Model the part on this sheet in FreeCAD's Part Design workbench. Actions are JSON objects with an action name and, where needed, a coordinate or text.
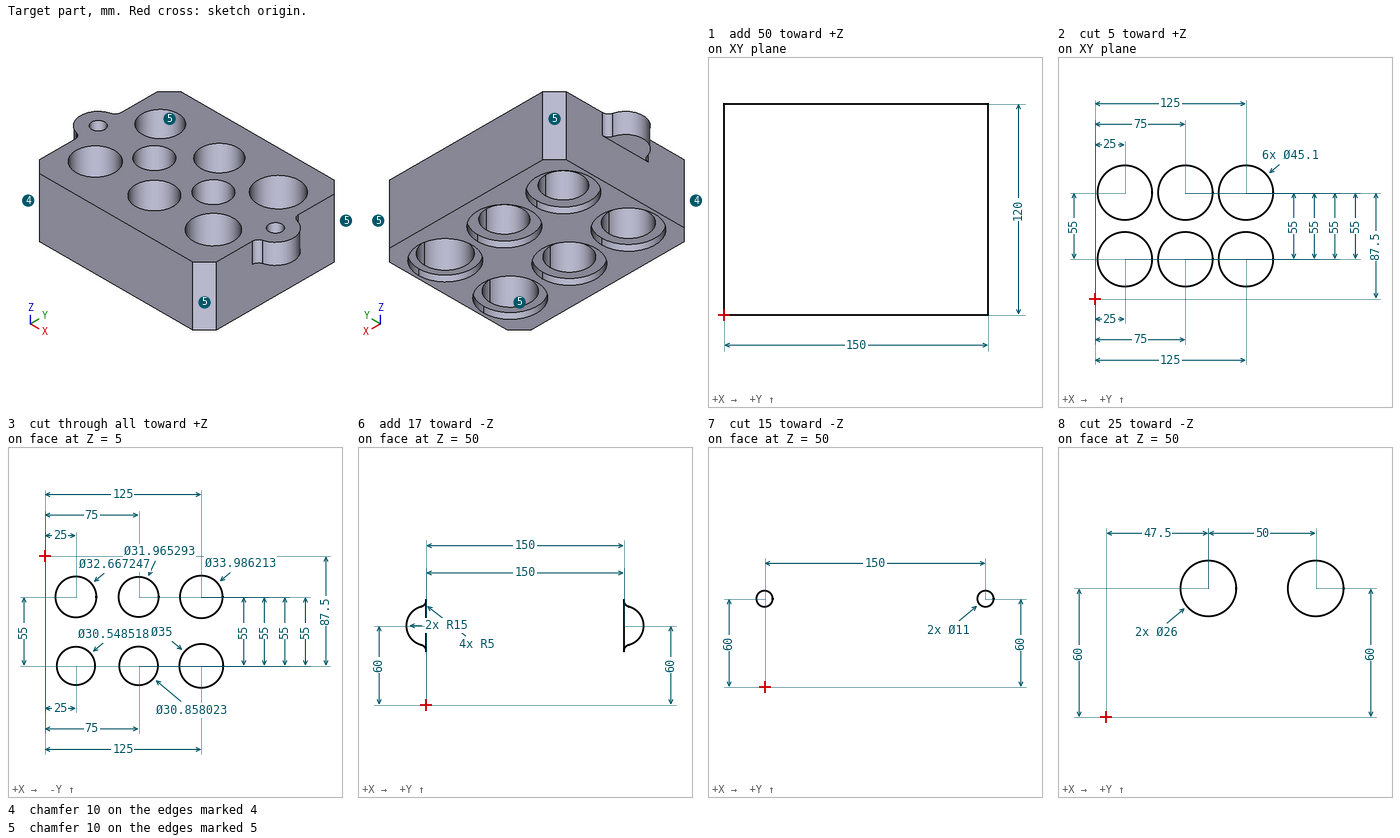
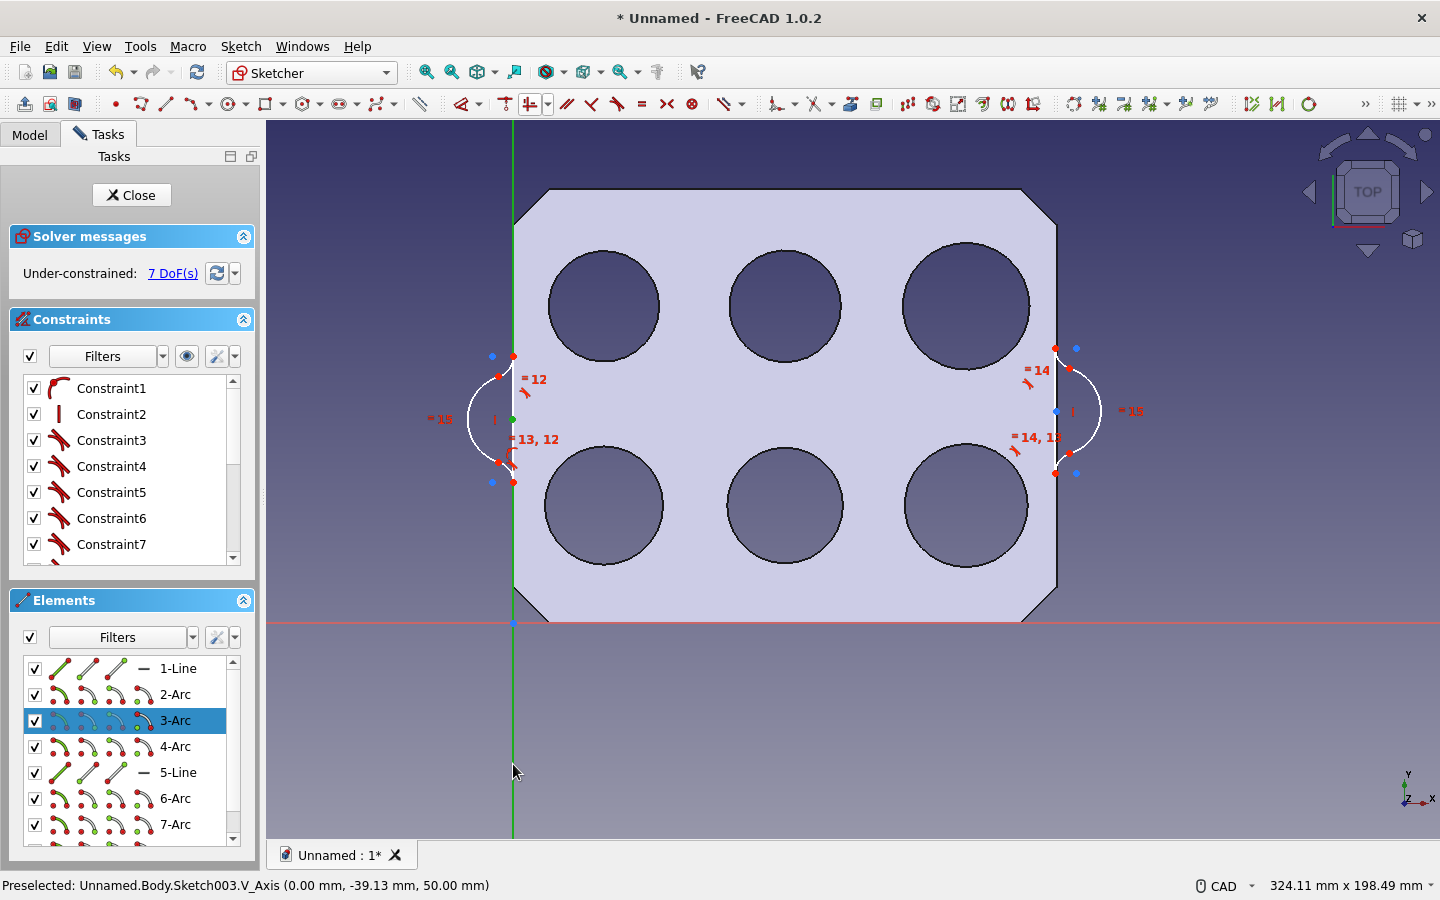
{"action": "left_click", "coordinate": [505, 104]}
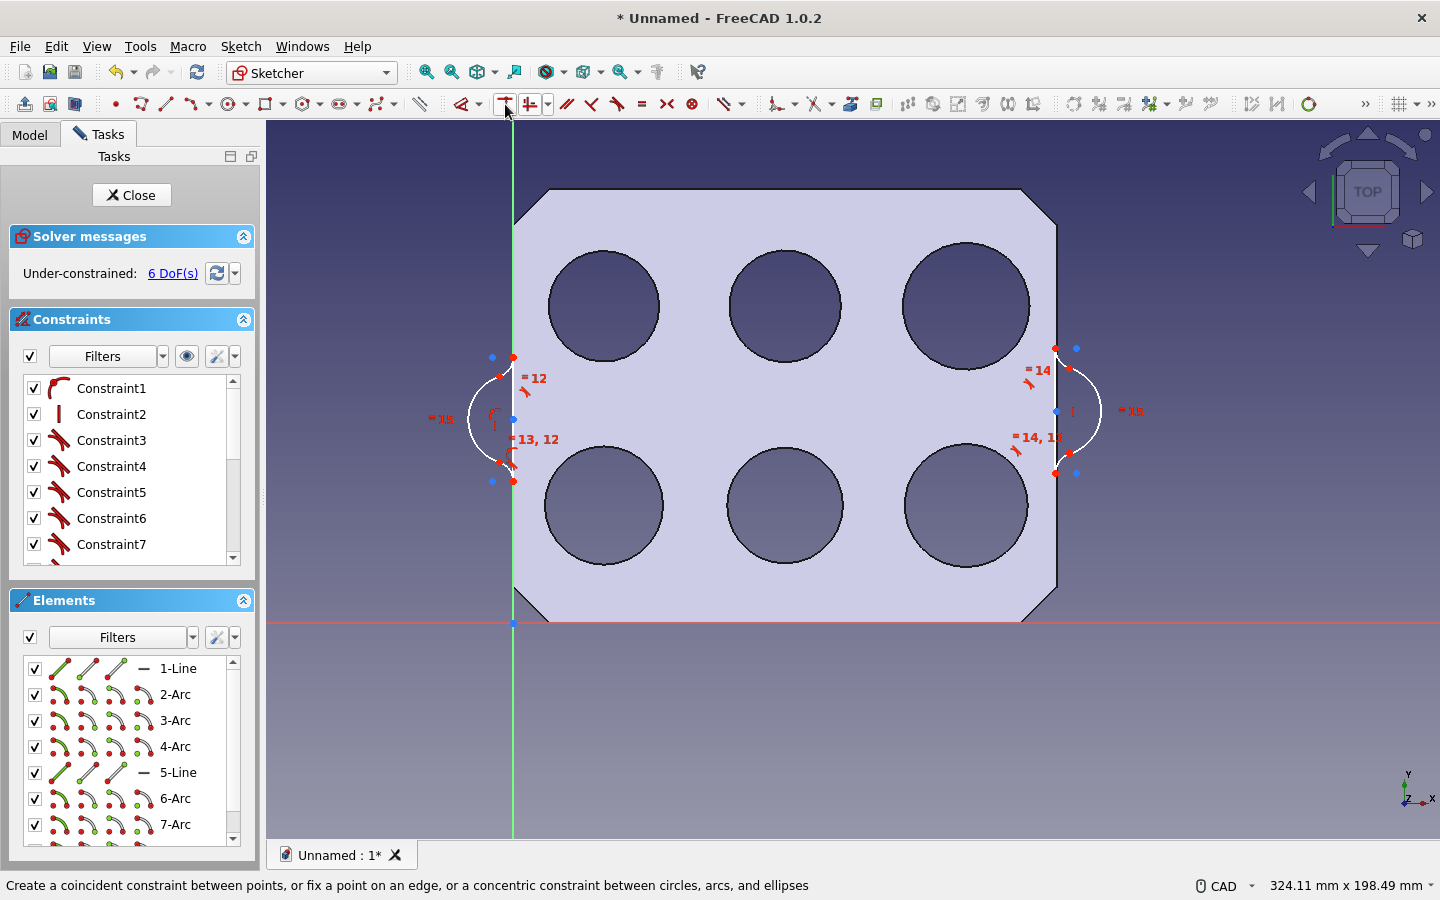
{"action": "key", "text": "d"}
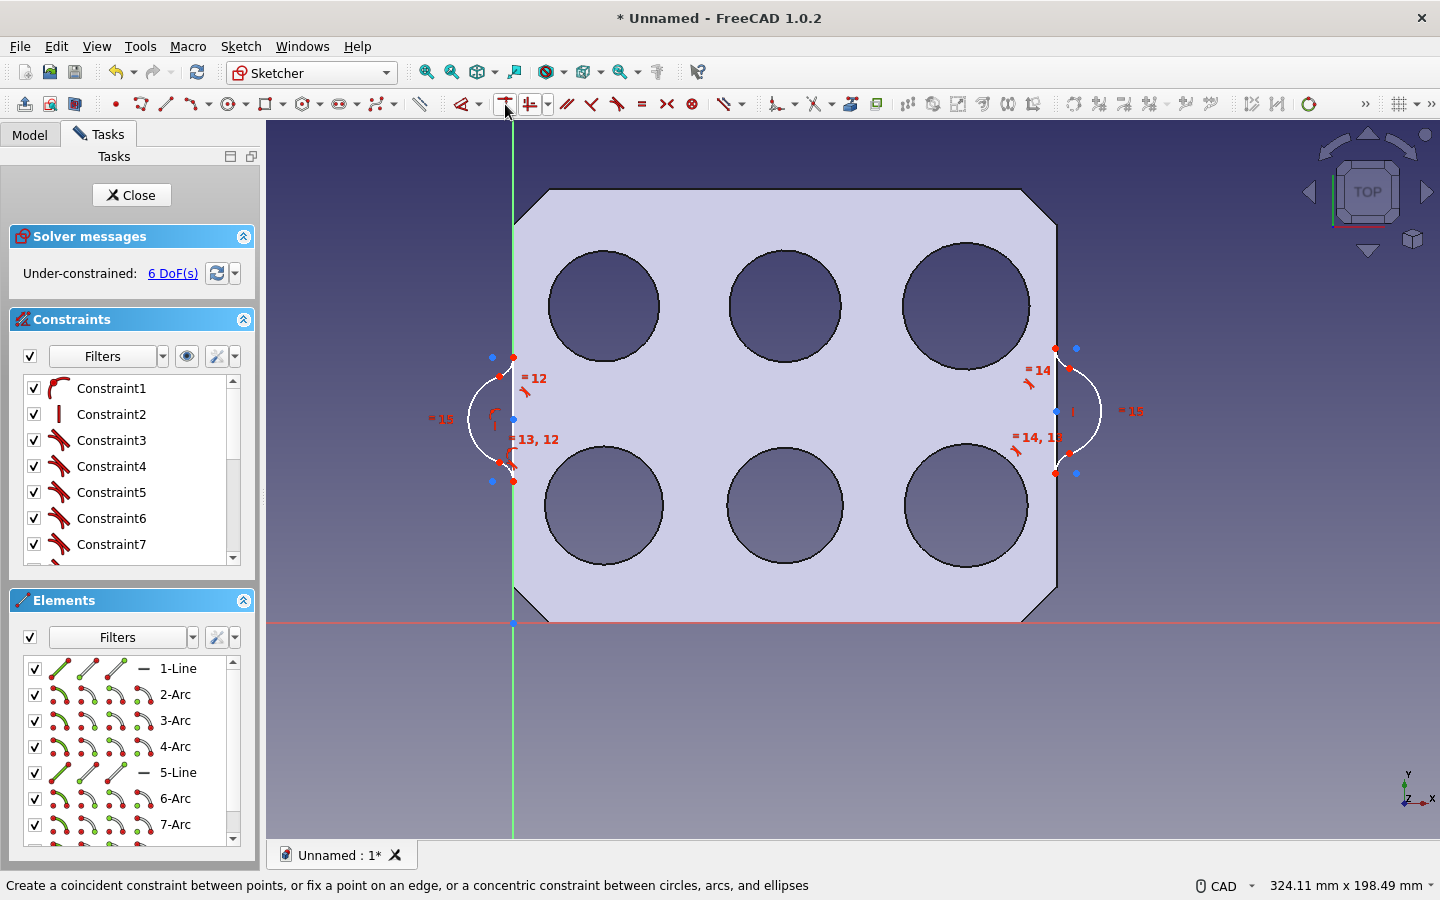
{"action": "scroll", "coordinate": [506, 373], "scroll_direction": "up", "scroll_amount": 4}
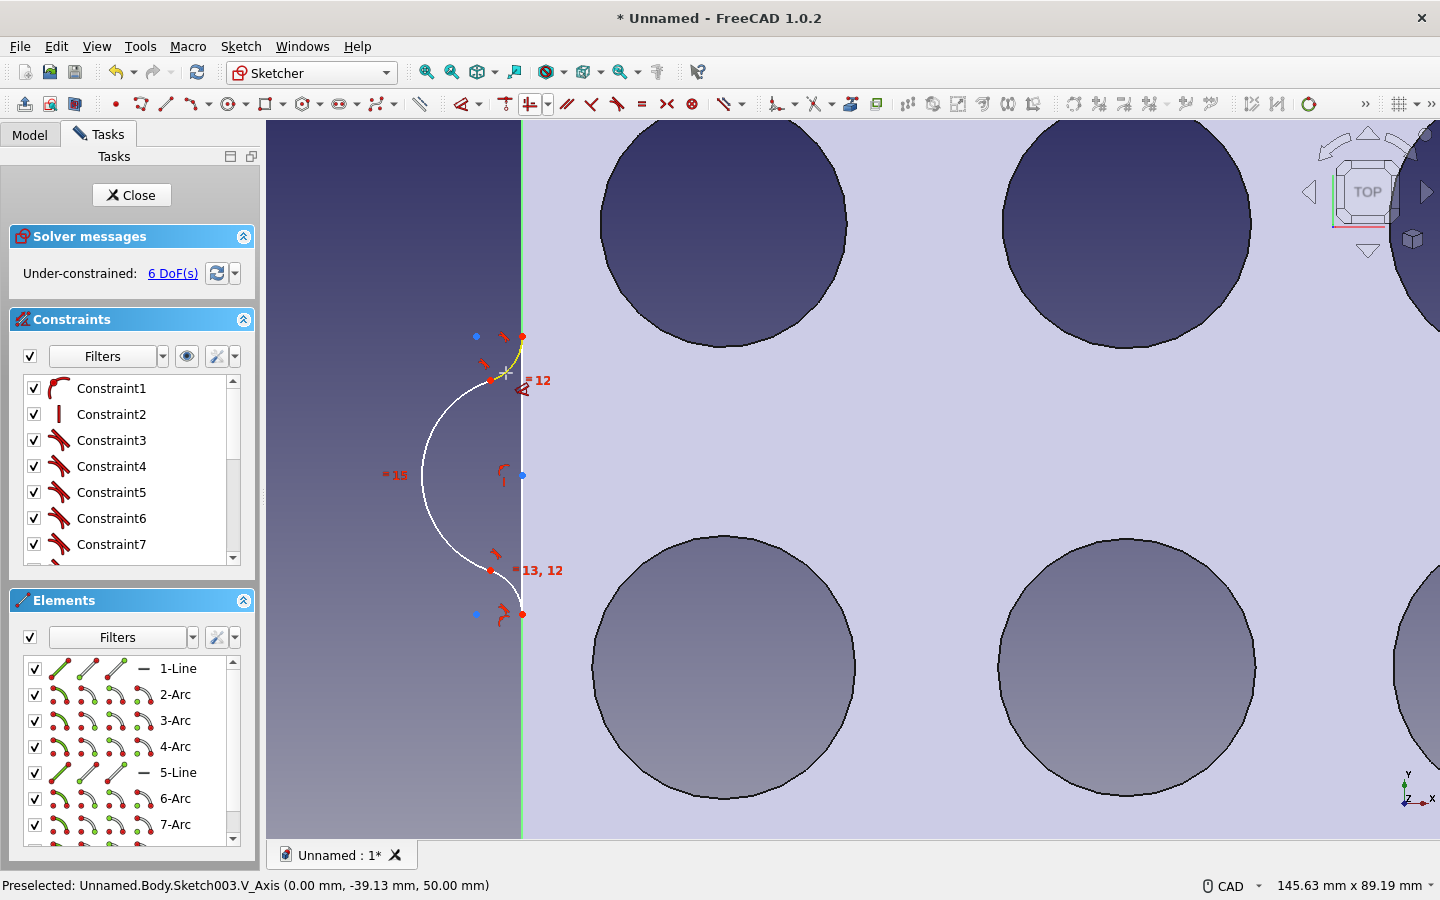
{"action": "left_click", "coordinate": [506, 372]}
{"action": "left_click", "coordinate": [492, 413]}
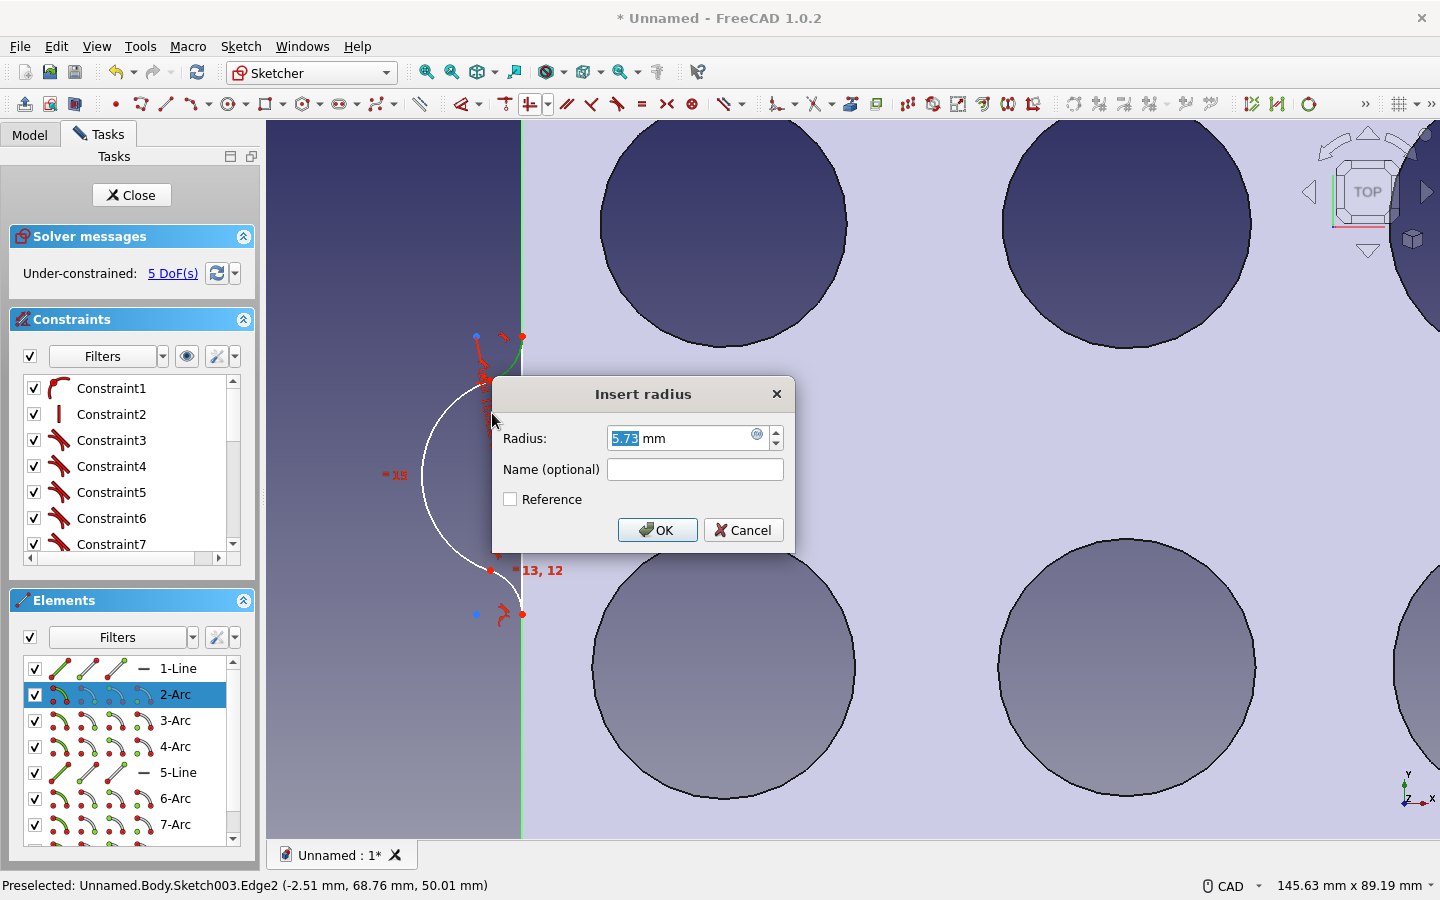
{"action": "type", "text": "5"}
{"action": "key", "text": "Return"}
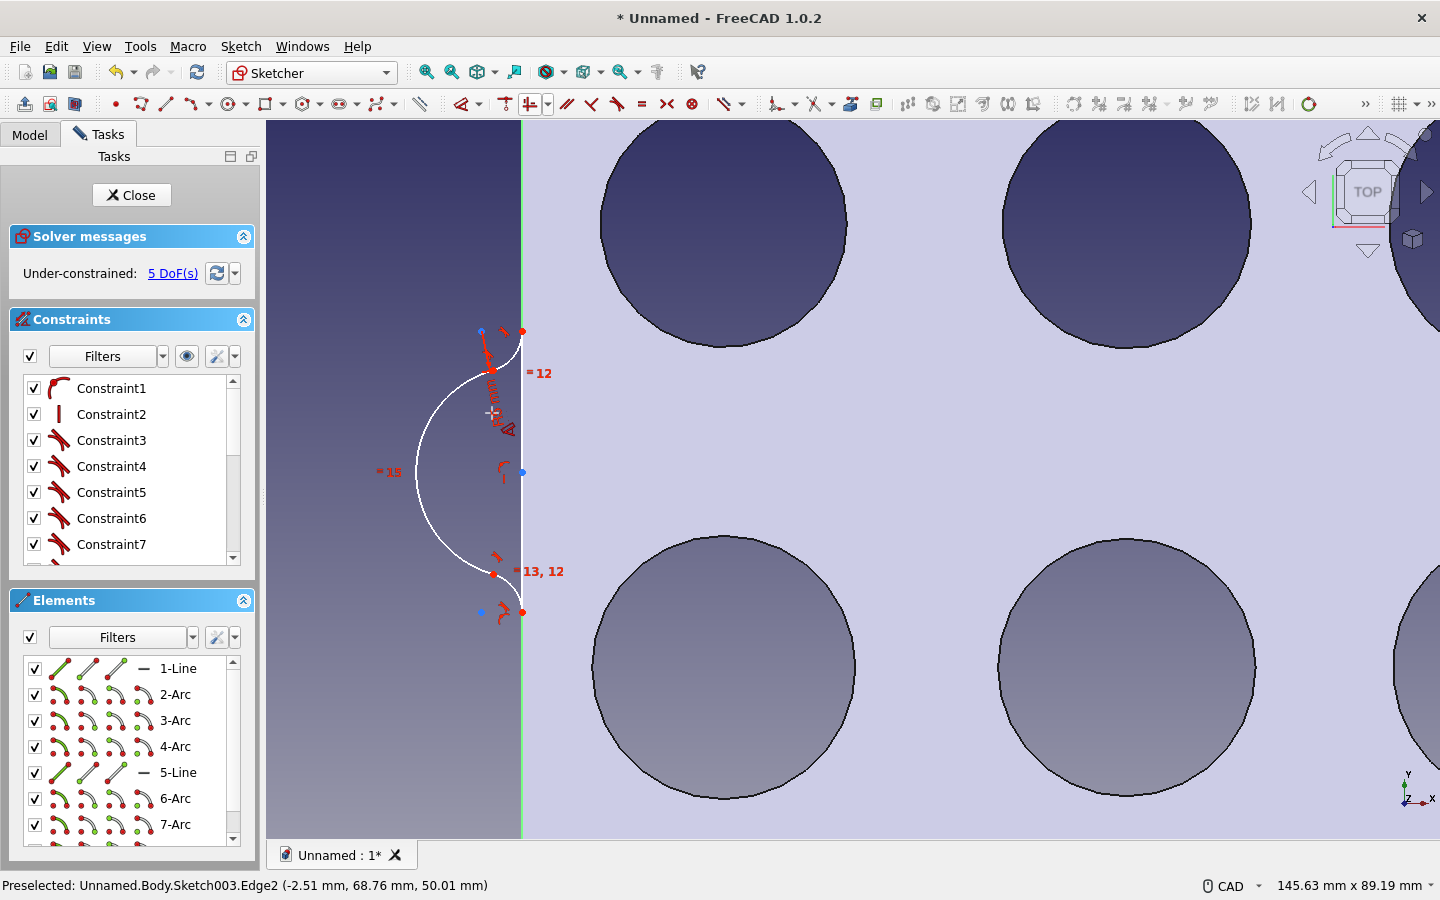
{"action": "left_click", "coordinate": [430, 420]}
{"action": "left_click", "coordinate": [402, 404]}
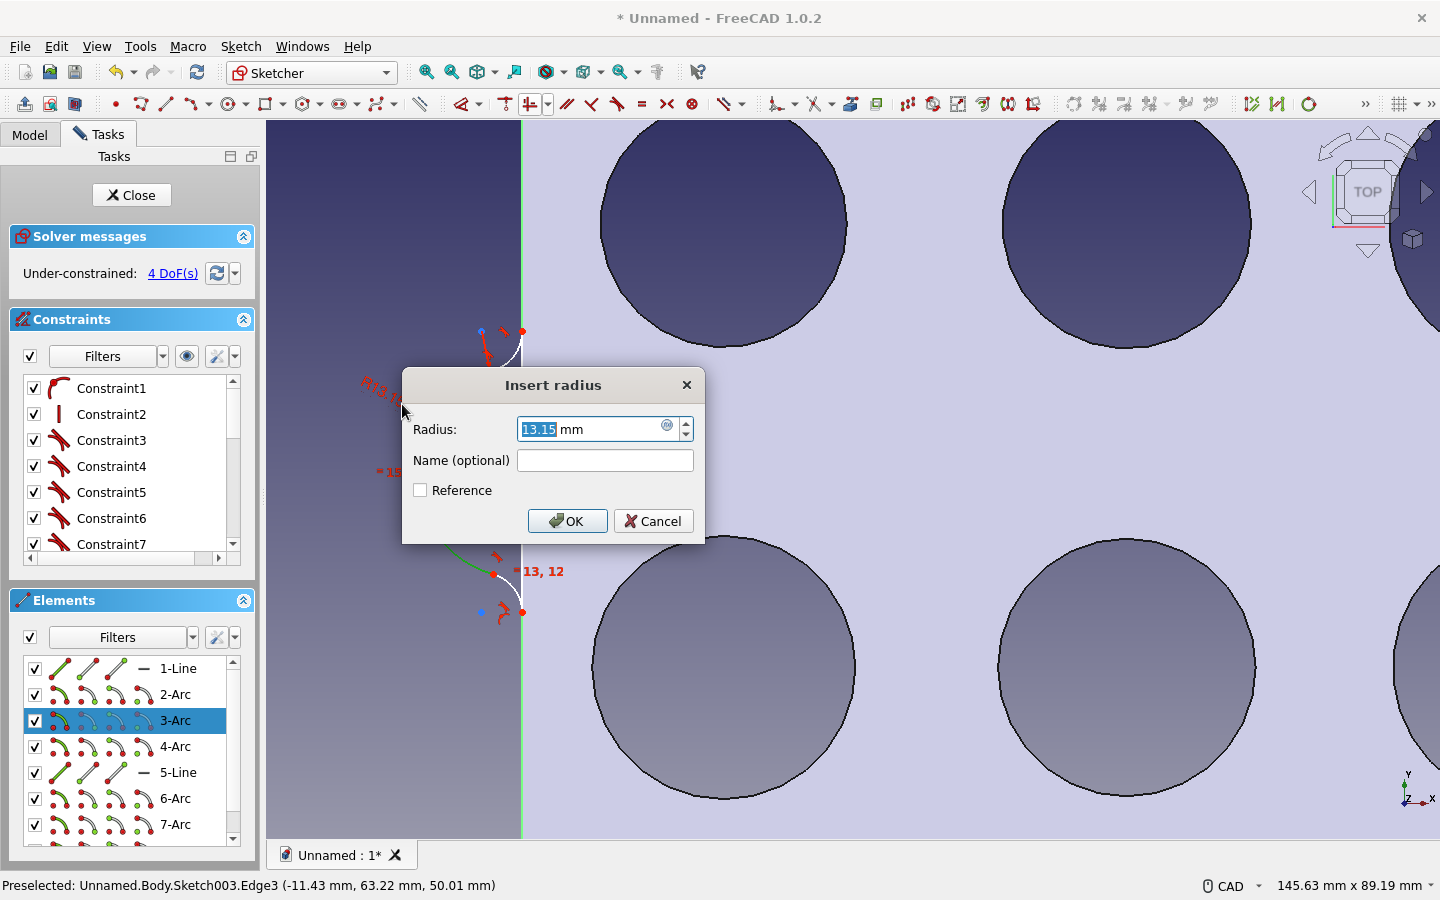
{"action": "type", "text": "15"}
{"action": "key", "text": "Return"}